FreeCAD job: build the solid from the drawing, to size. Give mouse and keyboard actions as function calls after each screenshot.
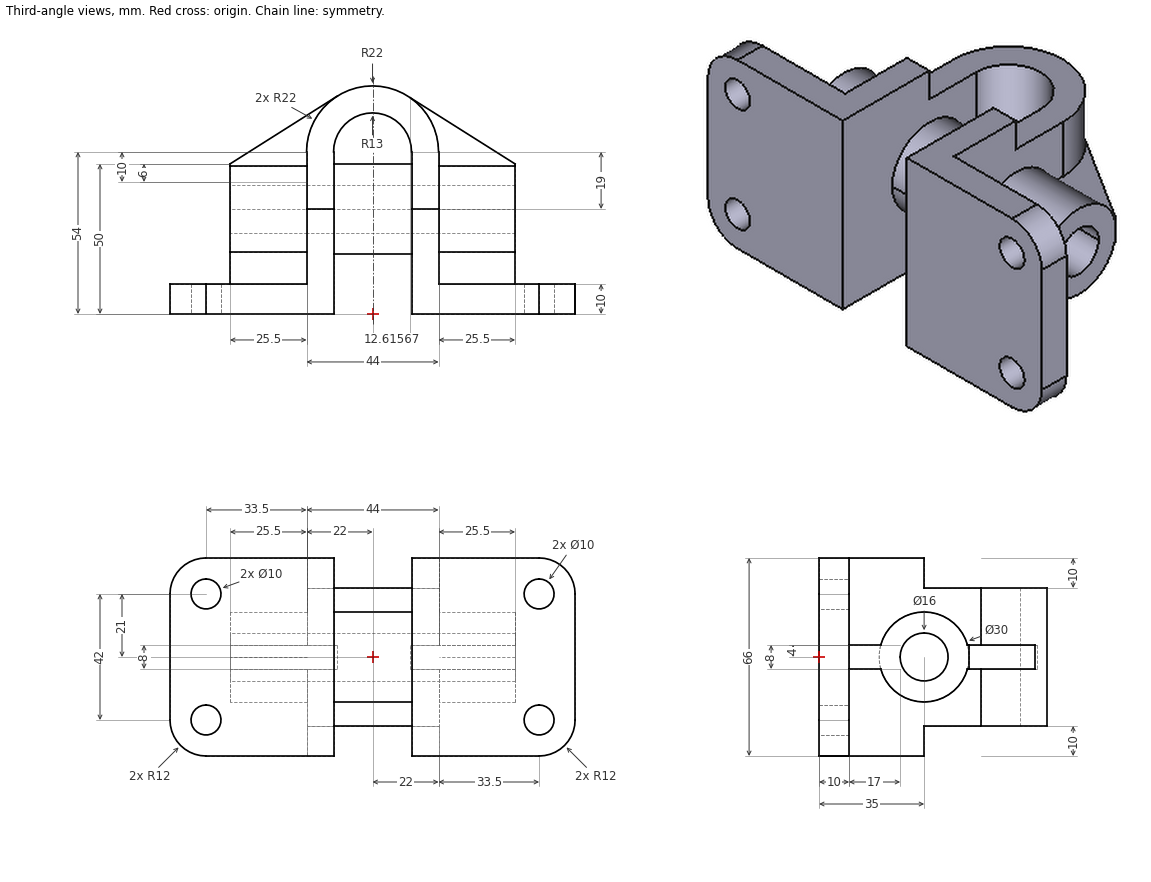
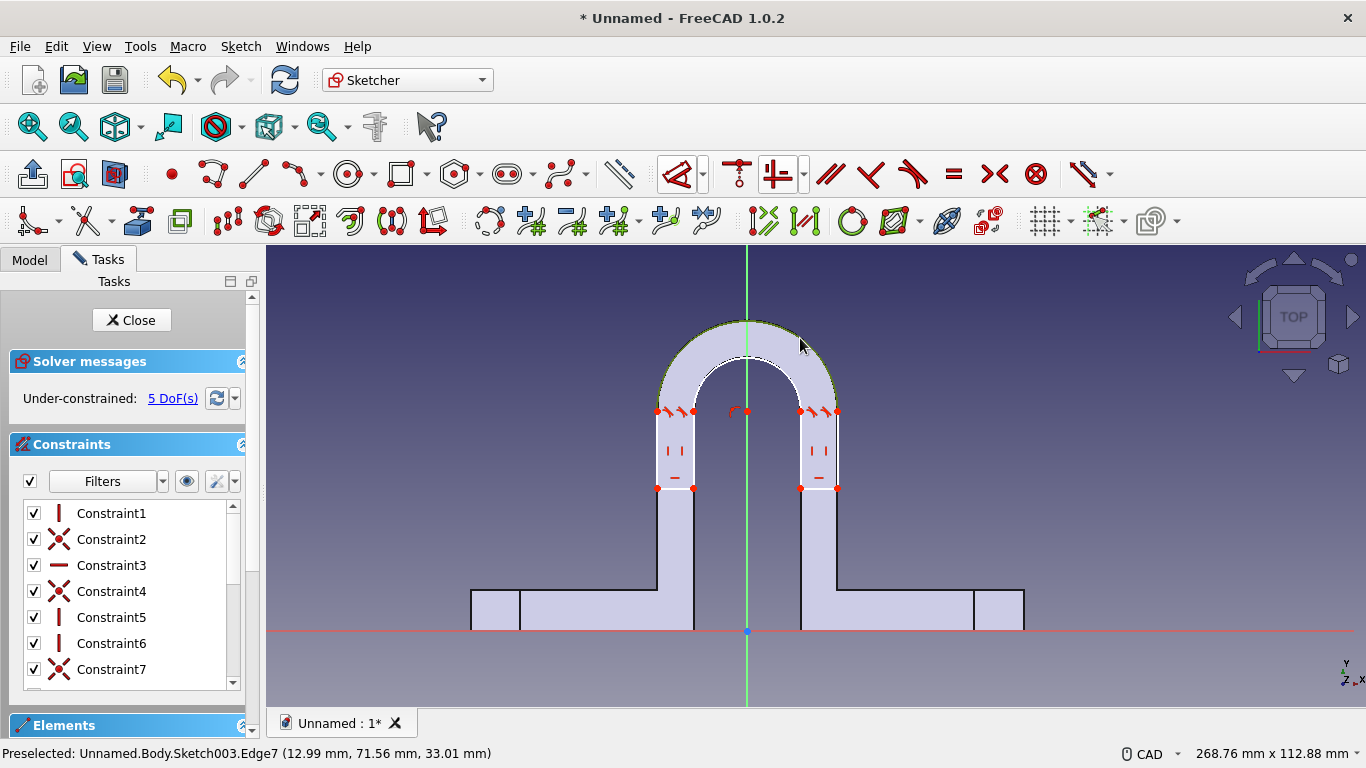
click(702, 174)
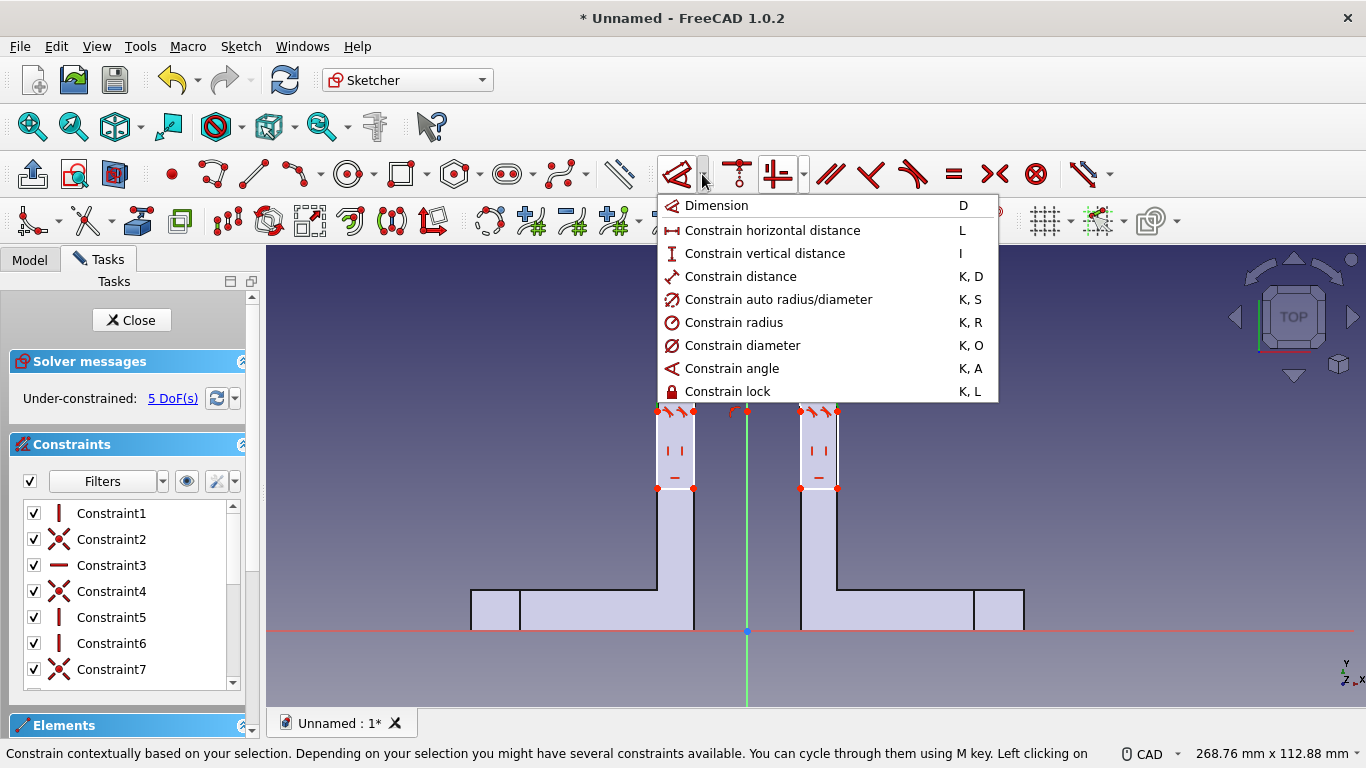
click(828, 322)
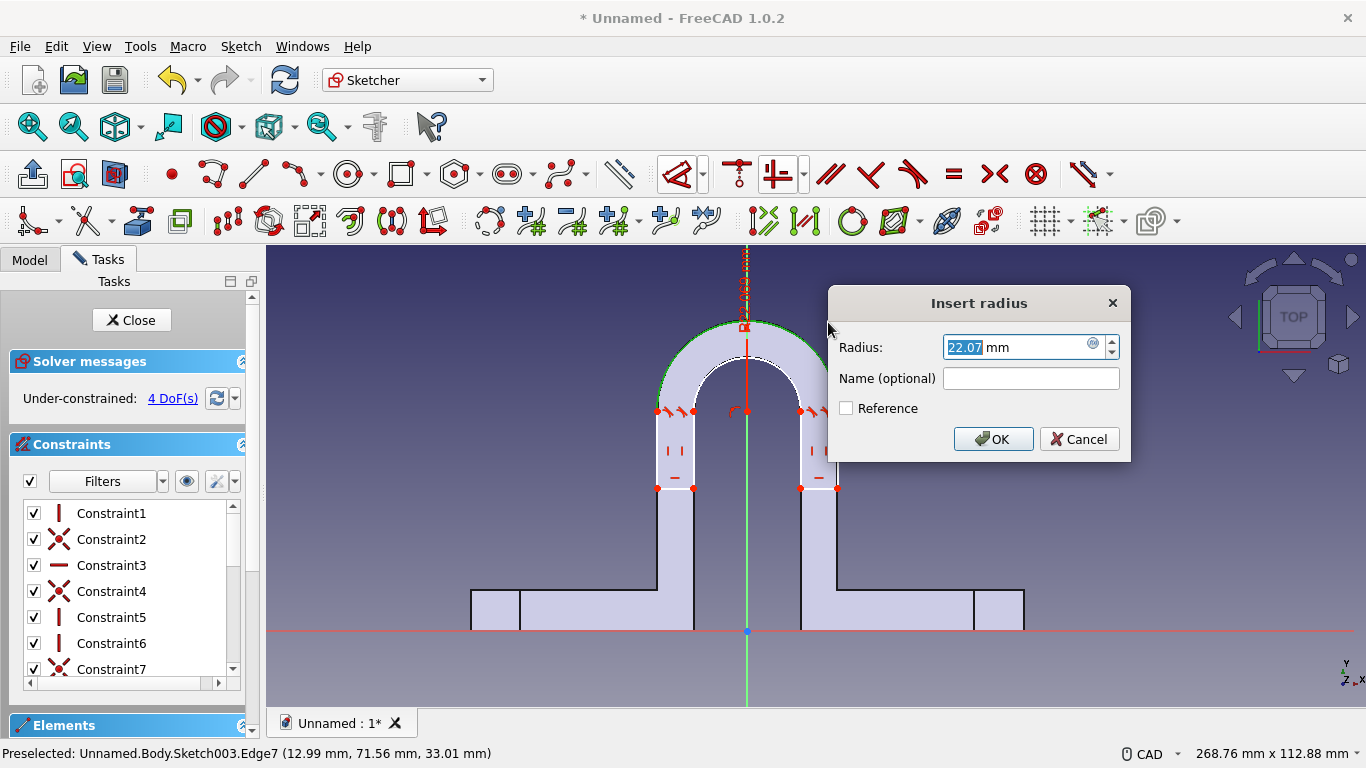
text(22)
key(Return)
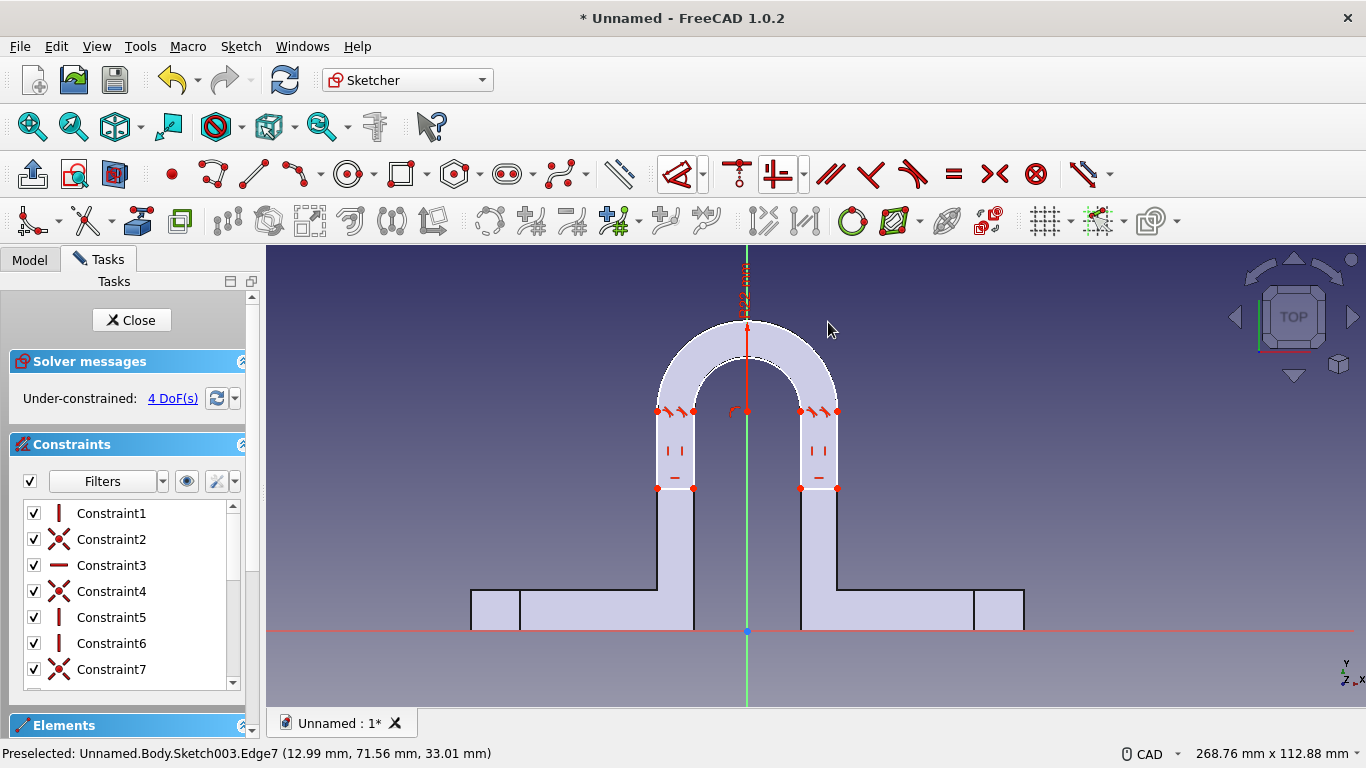
click(779, 368)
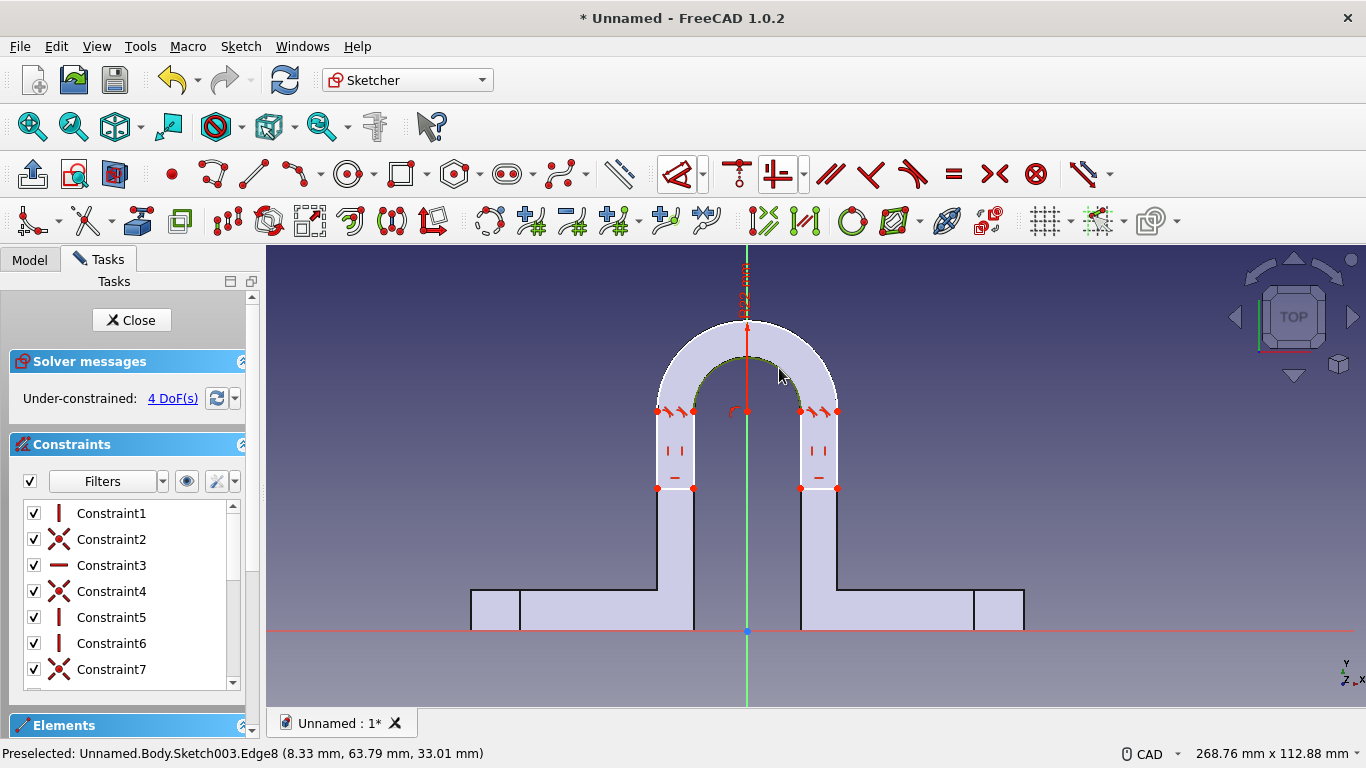
key(k)
key(r)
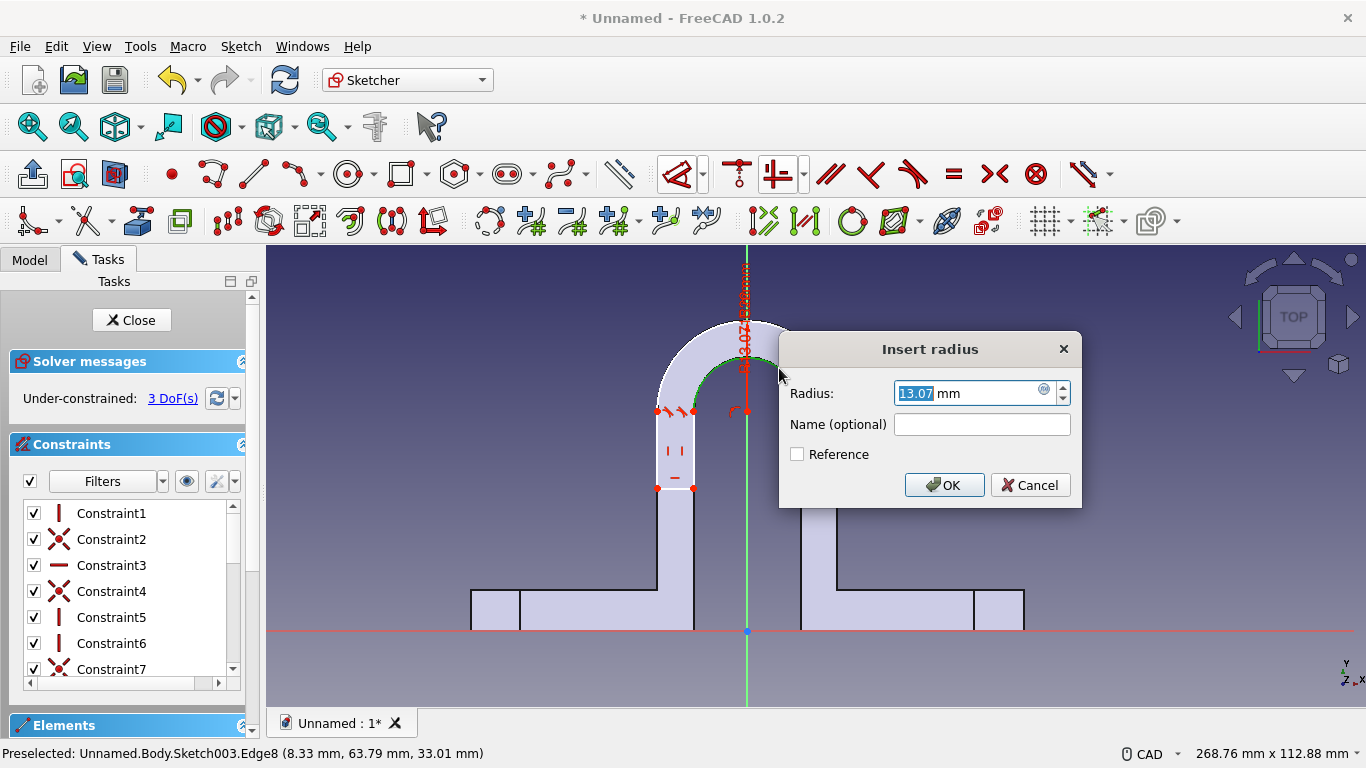
text(13)
key(Return)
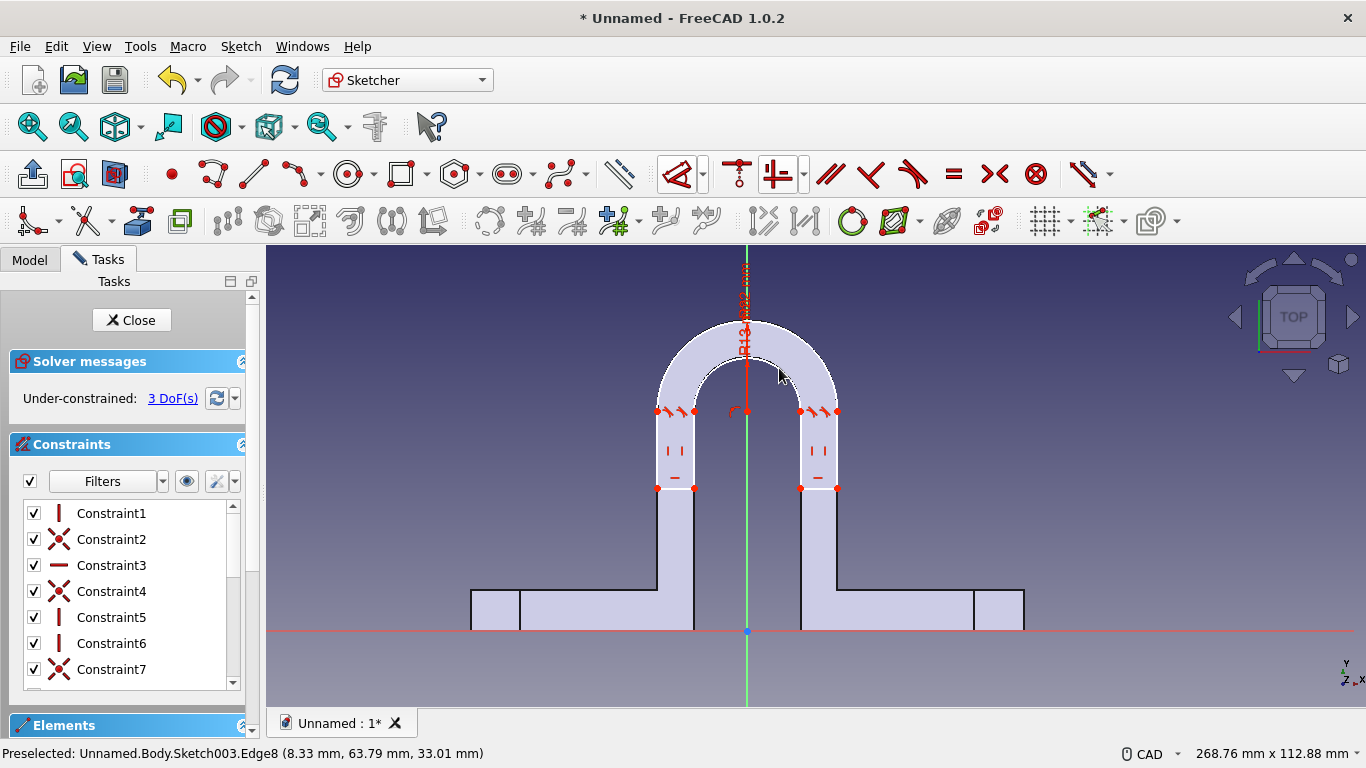
click(801, 435)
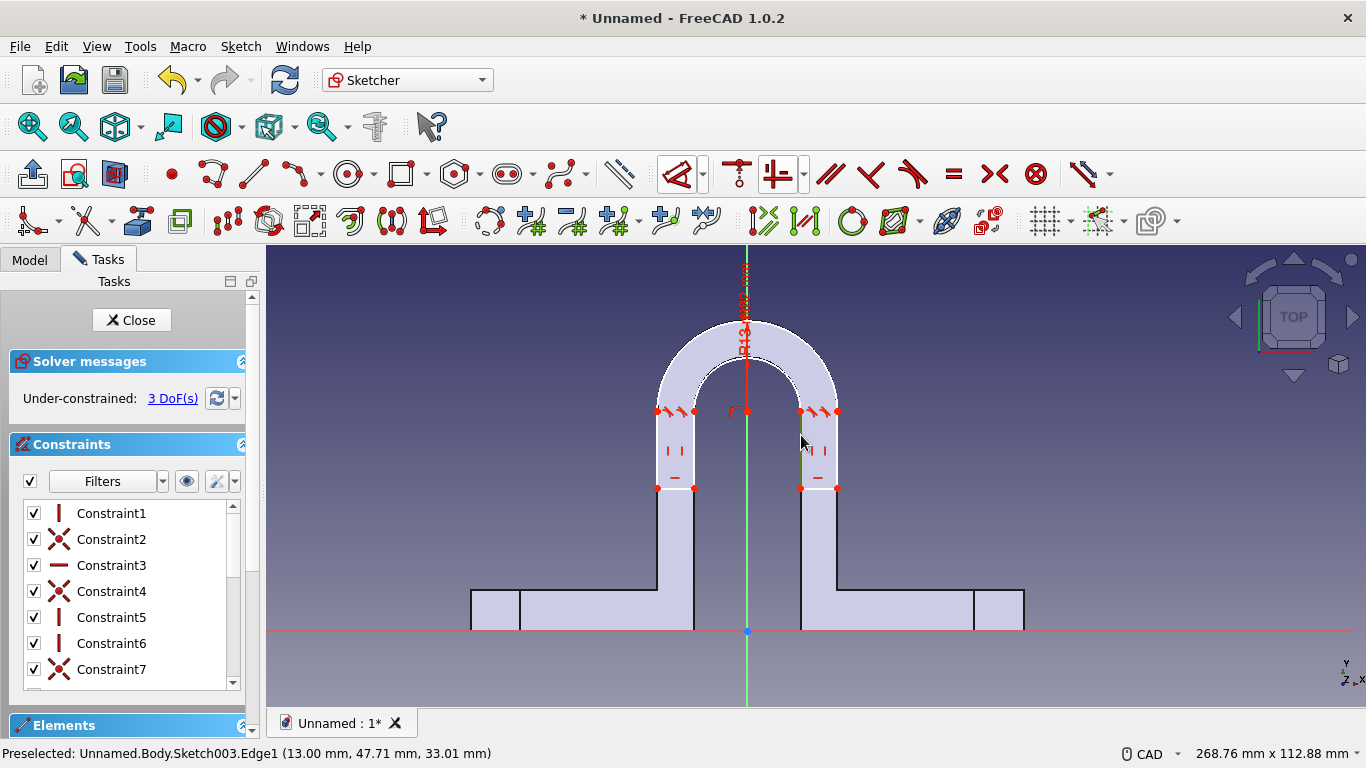
click(702, 174)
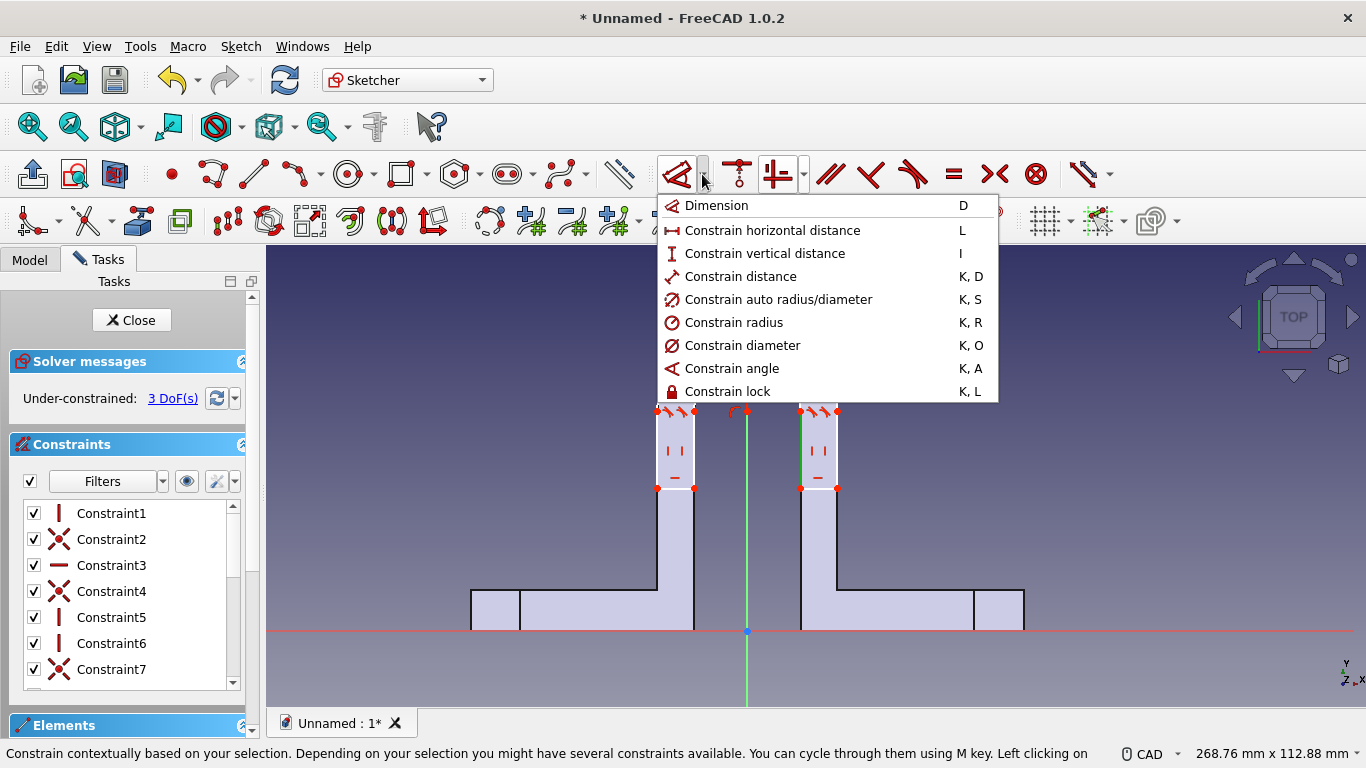
click(828, 254)